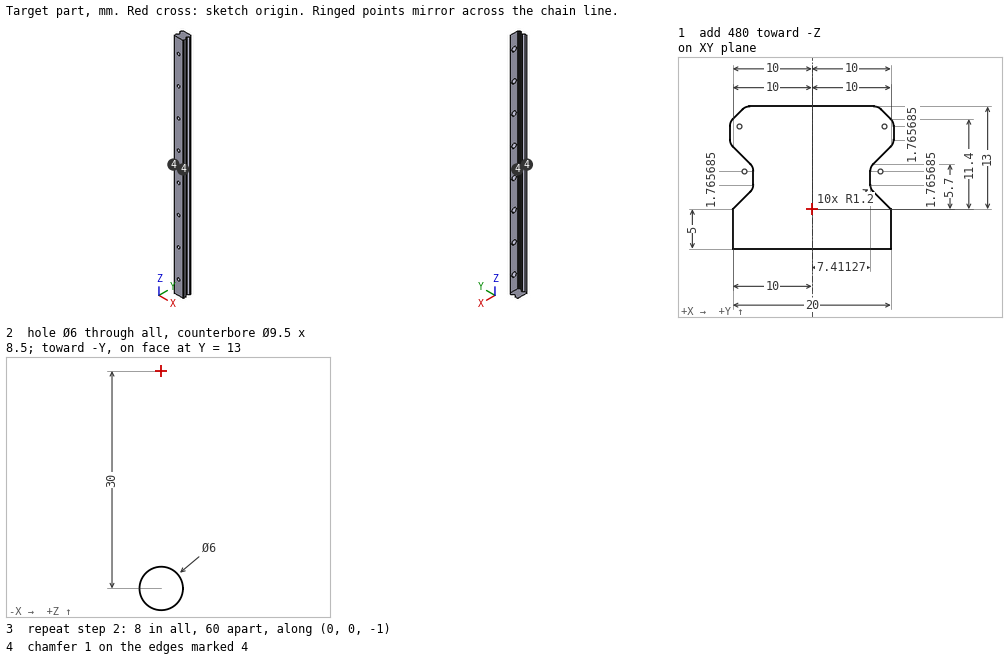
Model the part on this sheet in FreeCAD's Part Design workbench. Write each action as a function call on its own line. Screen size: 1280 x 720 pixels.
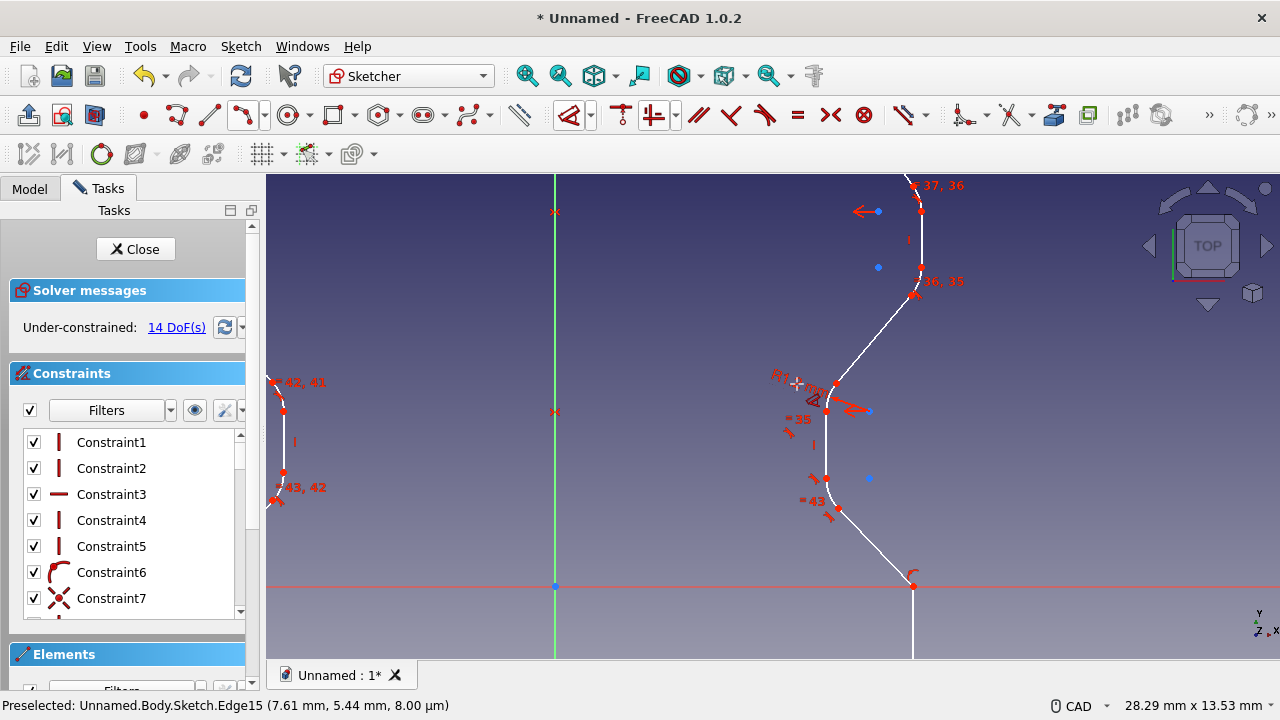
scroll(826, 395, down, 4)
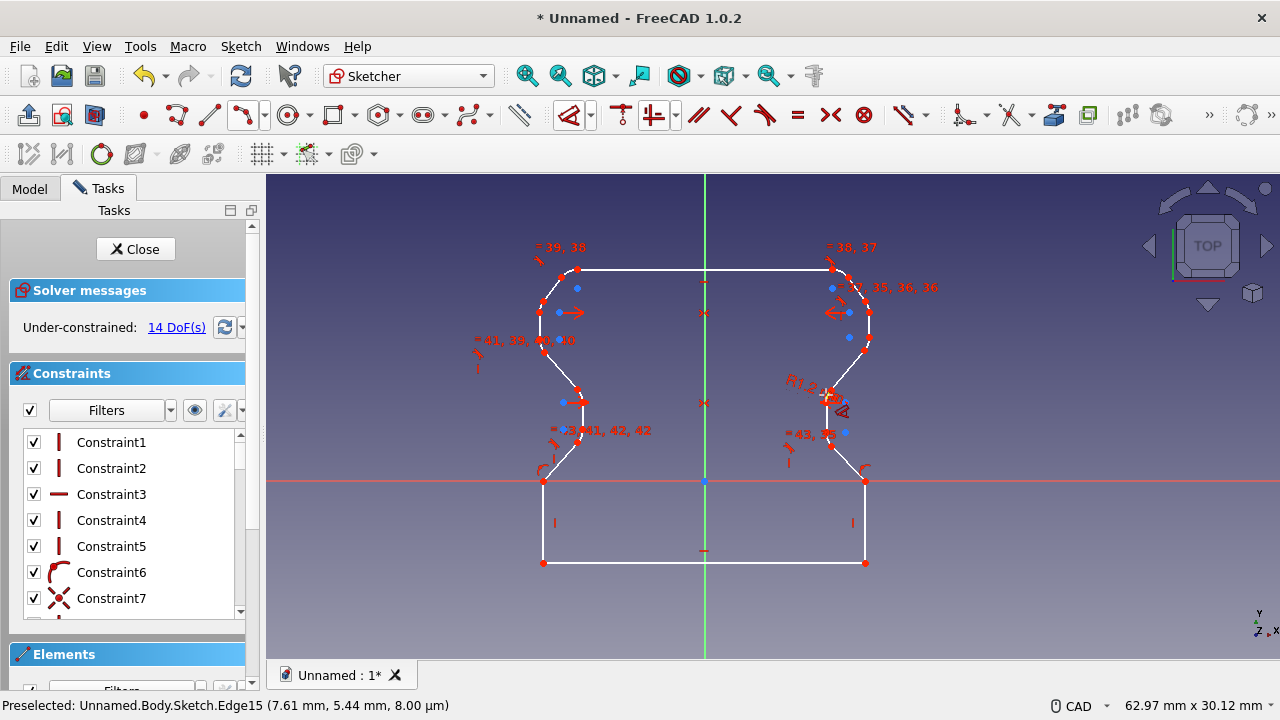
click(543, 506)
click(509, 522)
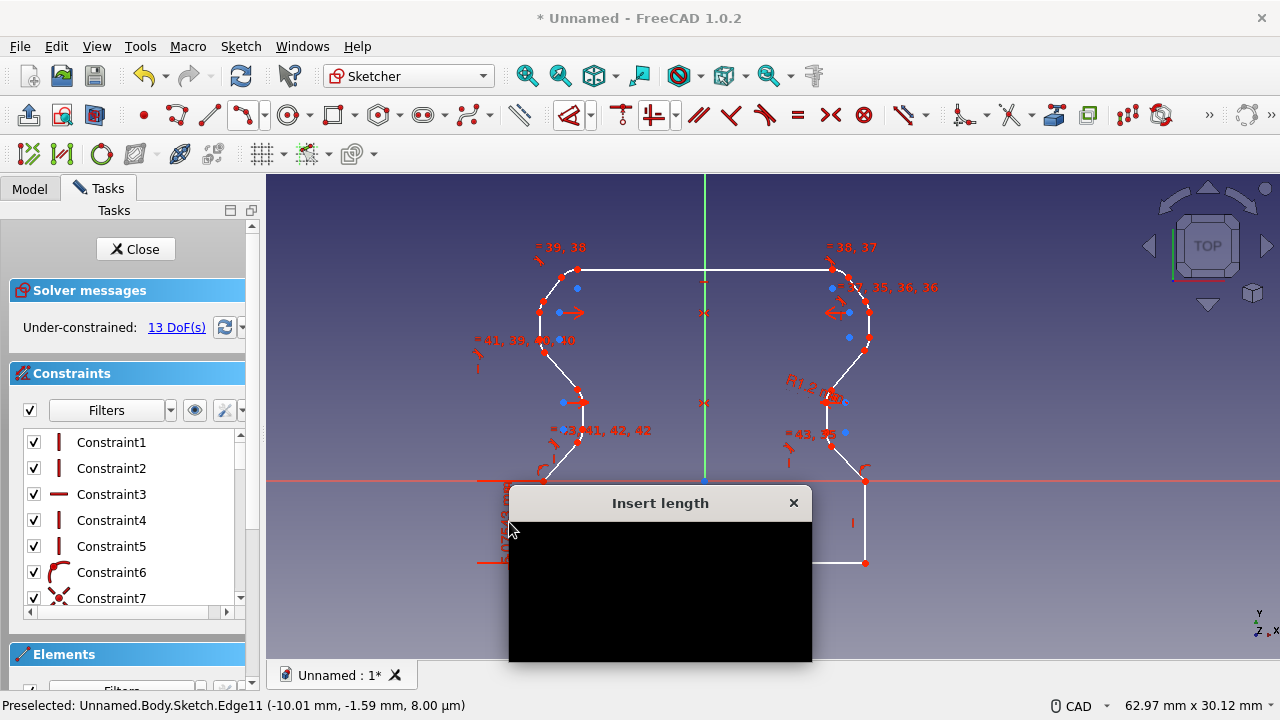
text(5)
key(Return)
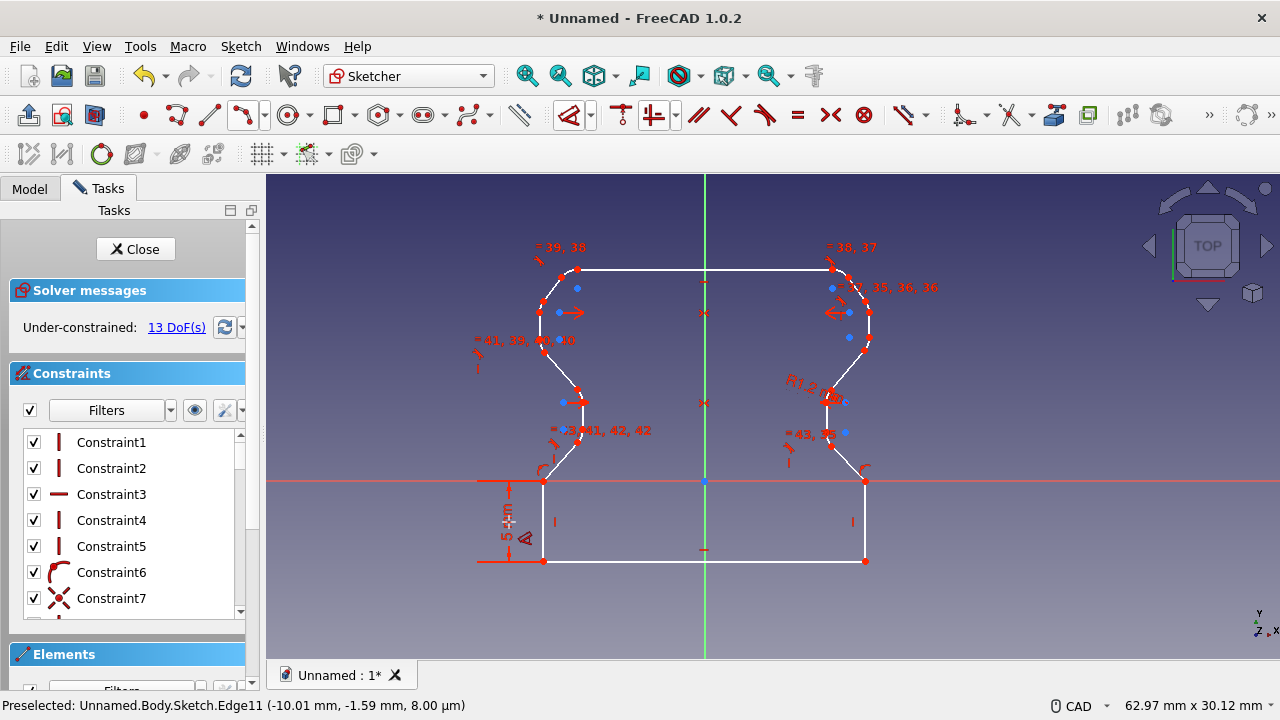
click(640, 562)
click(630, 596)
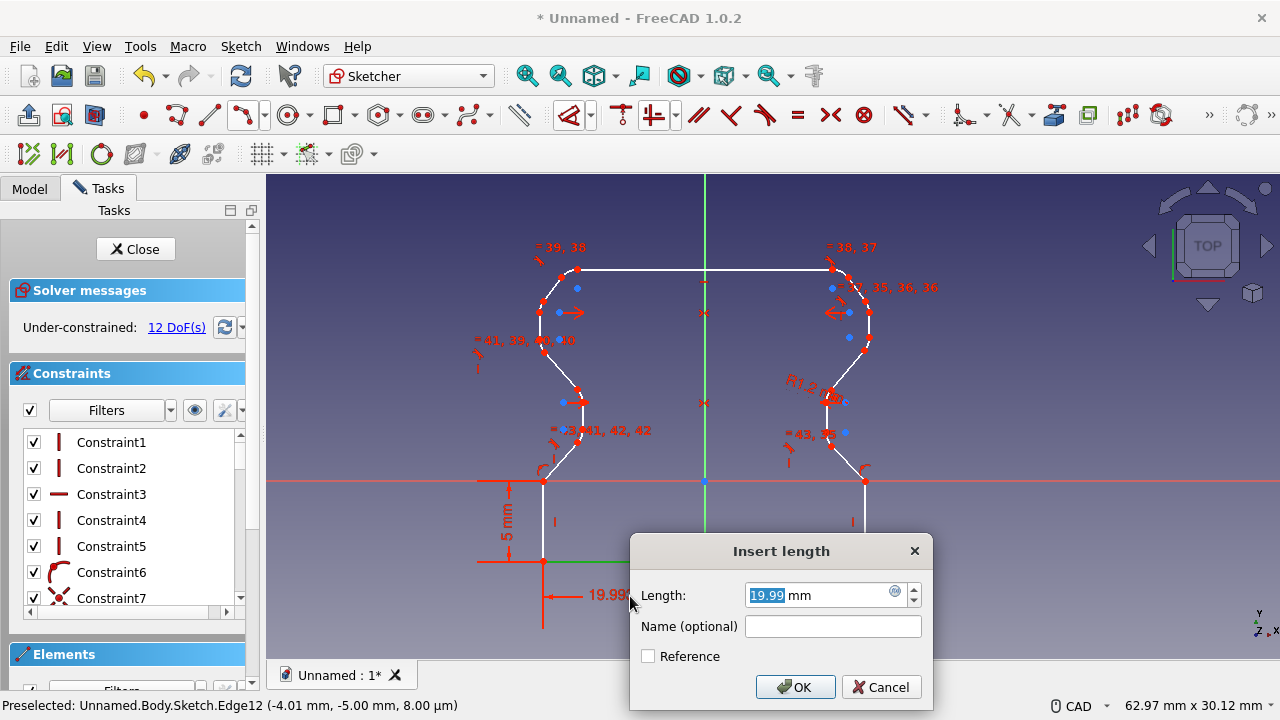
text(20)
key(Return)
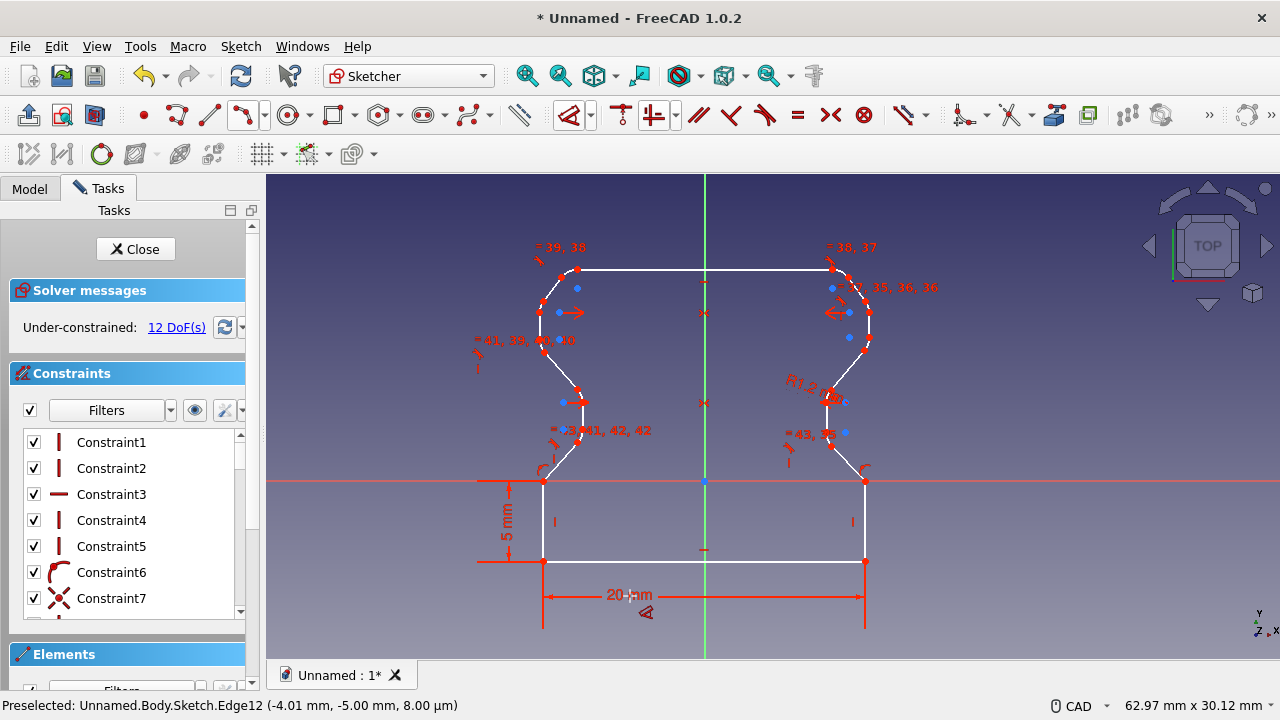
click(865, 350)
click(785, 316)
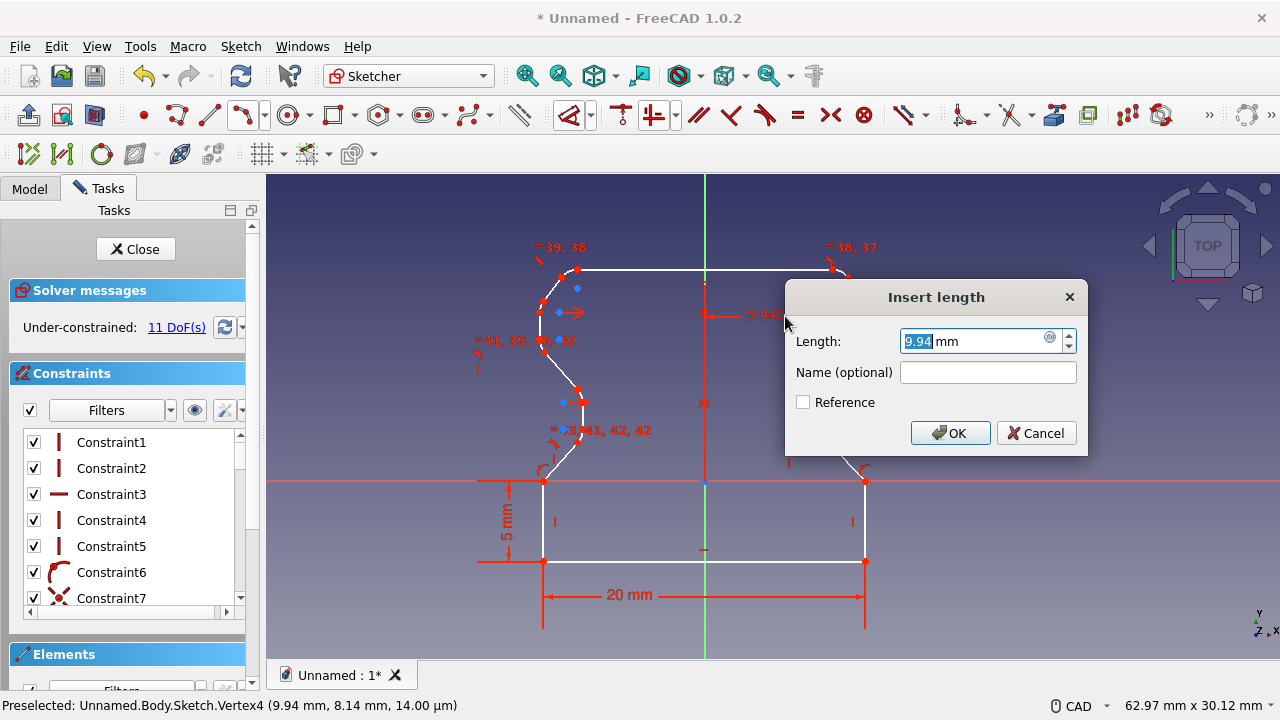
text(10)
key(Return)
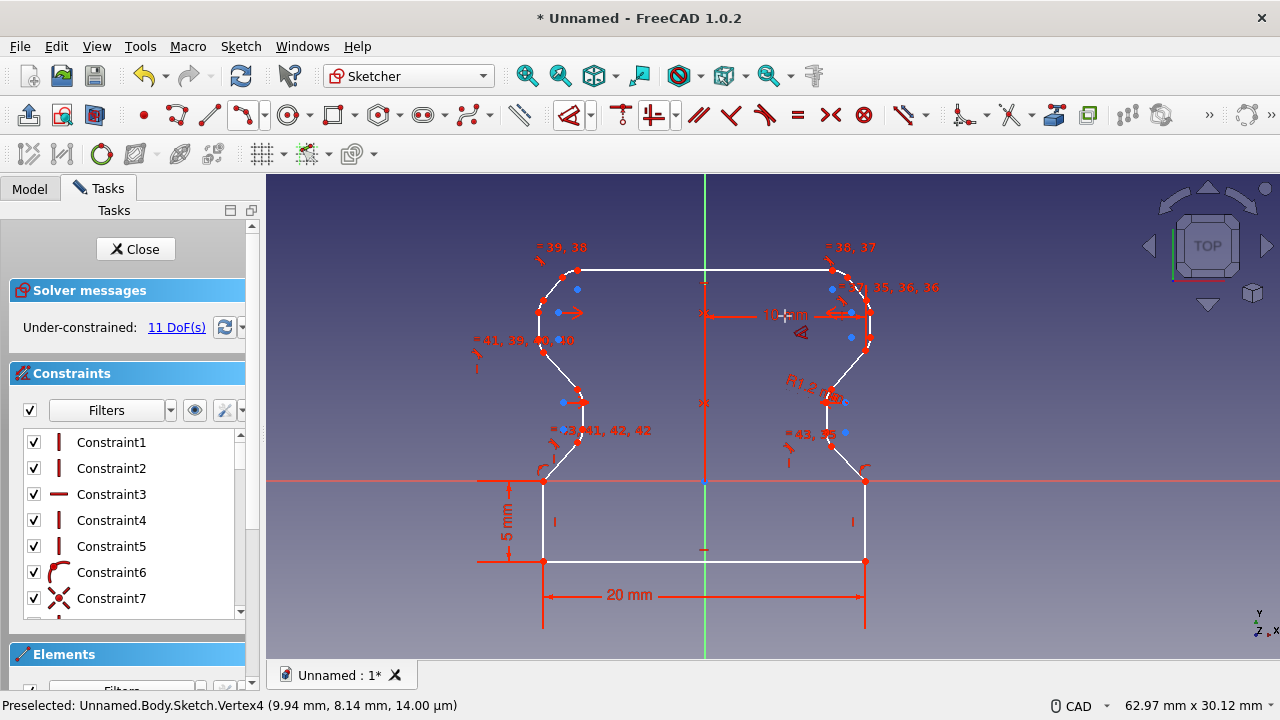
click(866, 301)
click(785, 515)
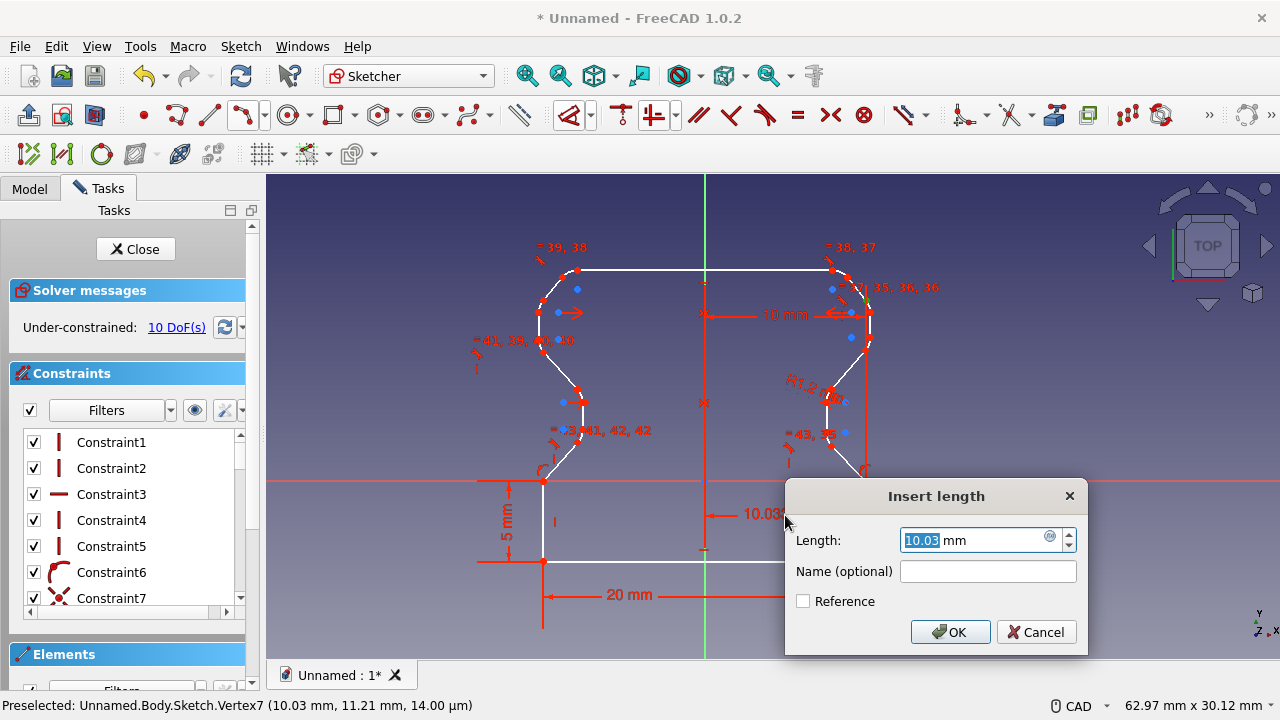
text(10)
key(Return)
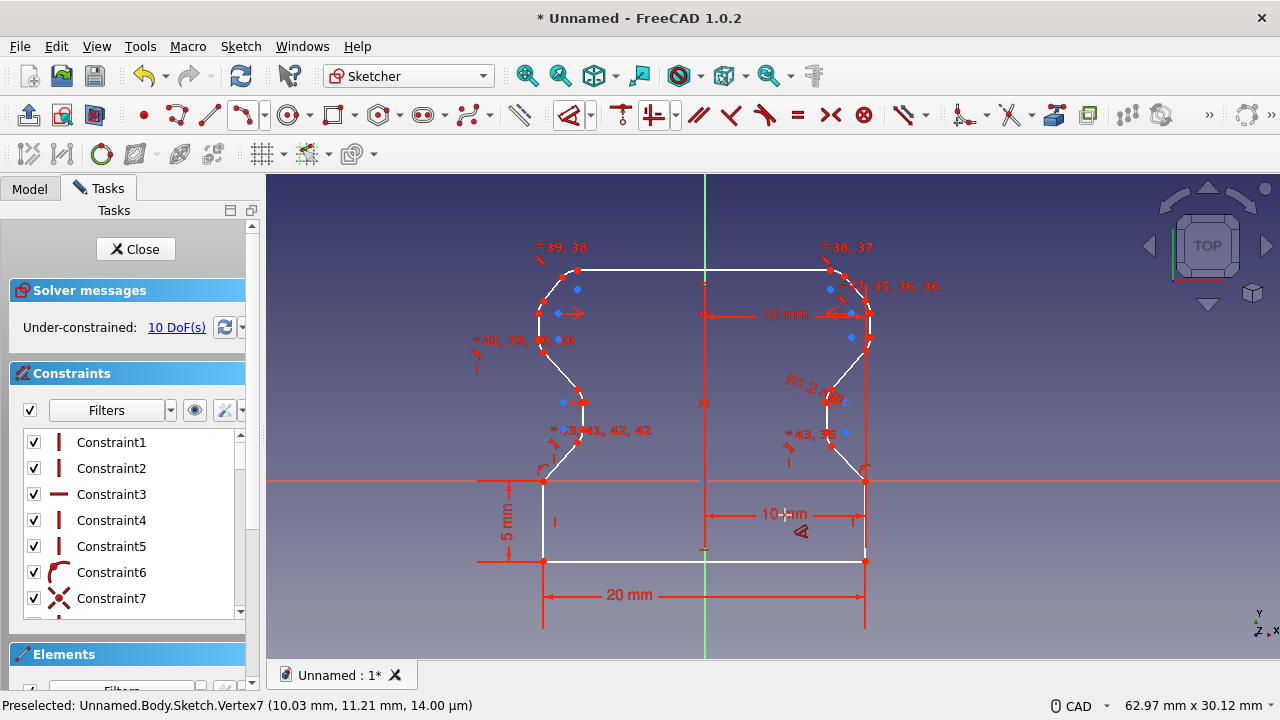
click(830, 270)
click(864, 424)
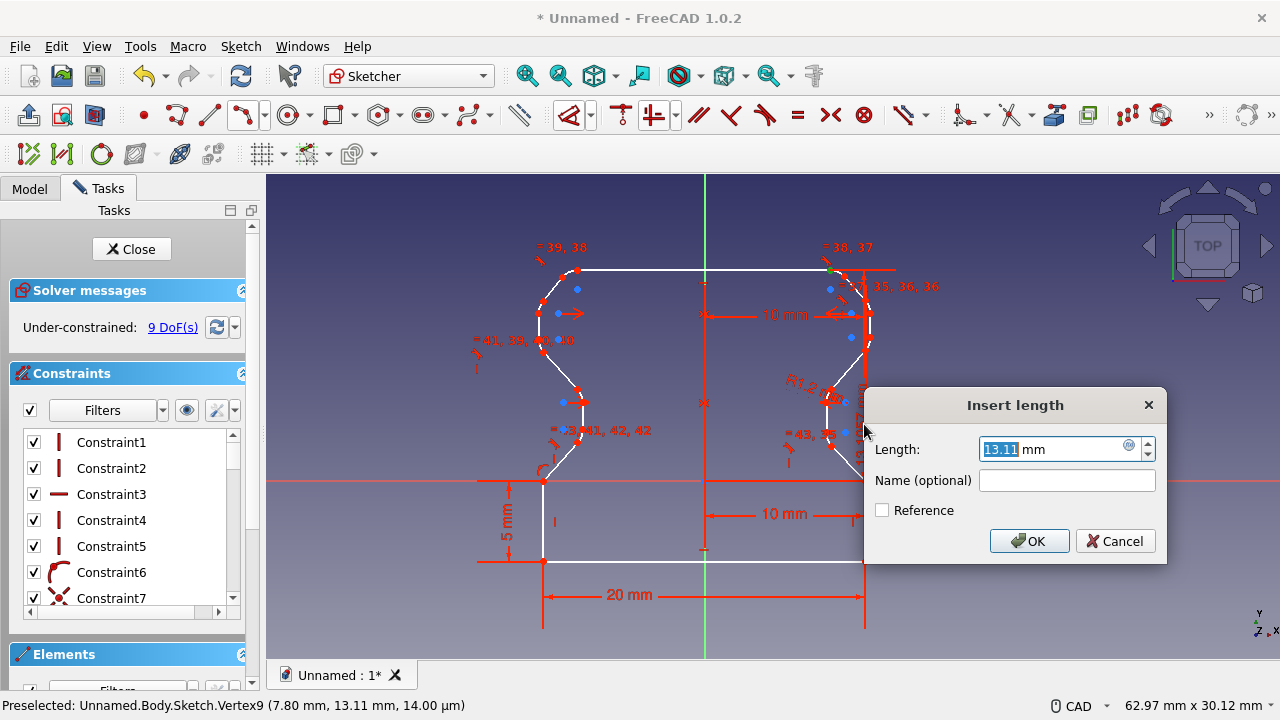
text(13)
key(Return)